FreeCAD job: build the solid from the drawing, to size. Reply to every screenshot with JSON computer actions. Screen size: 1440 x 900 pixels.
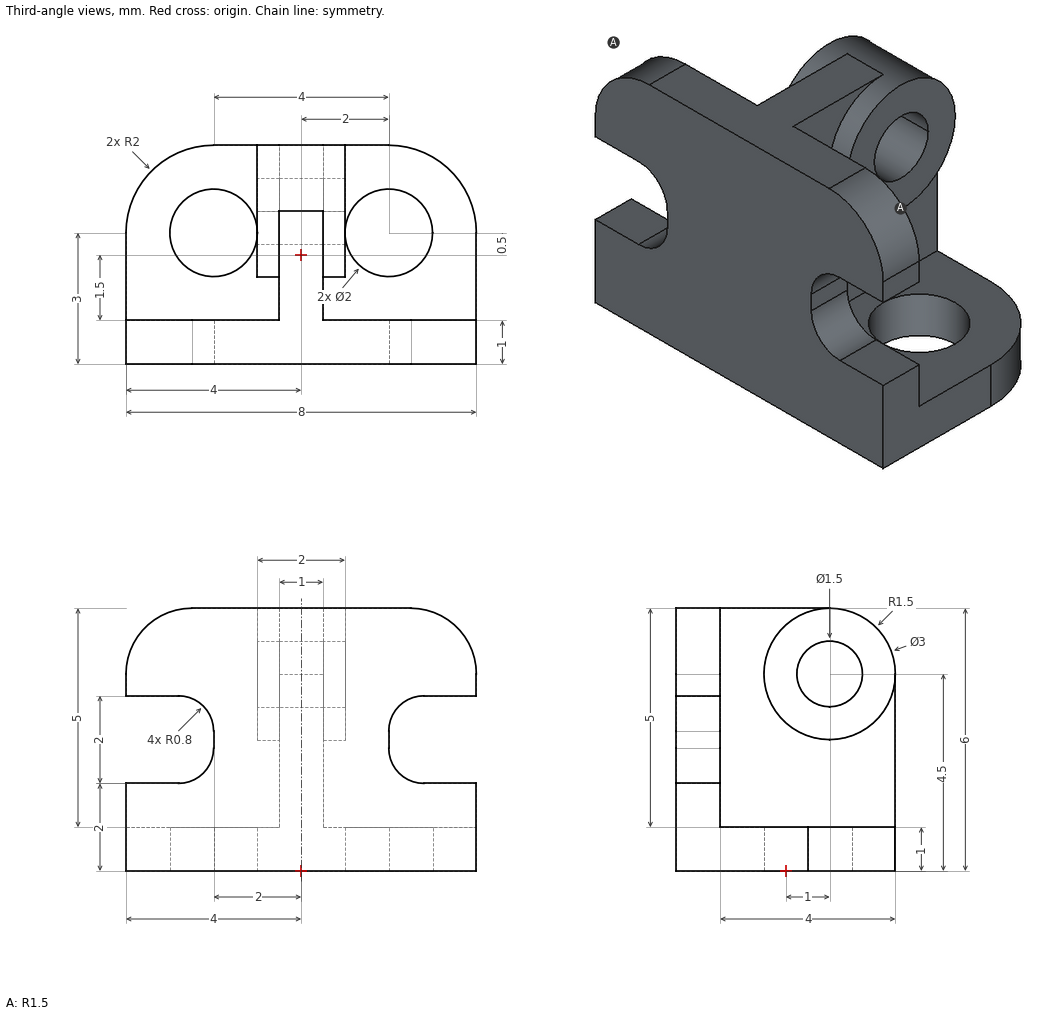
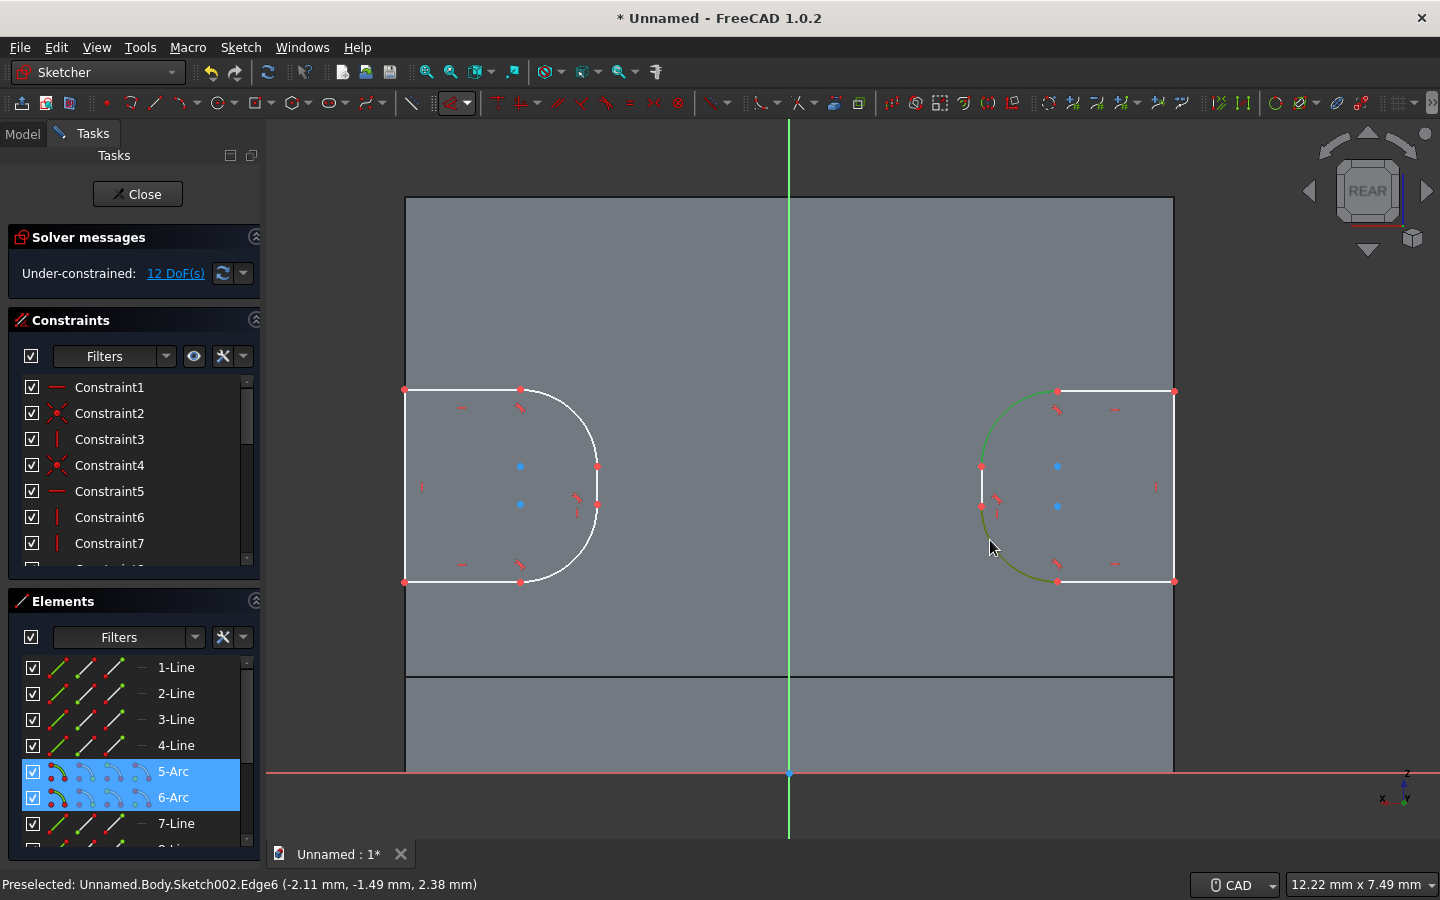
{"action": "left_click", "coordinate": [589, 432]}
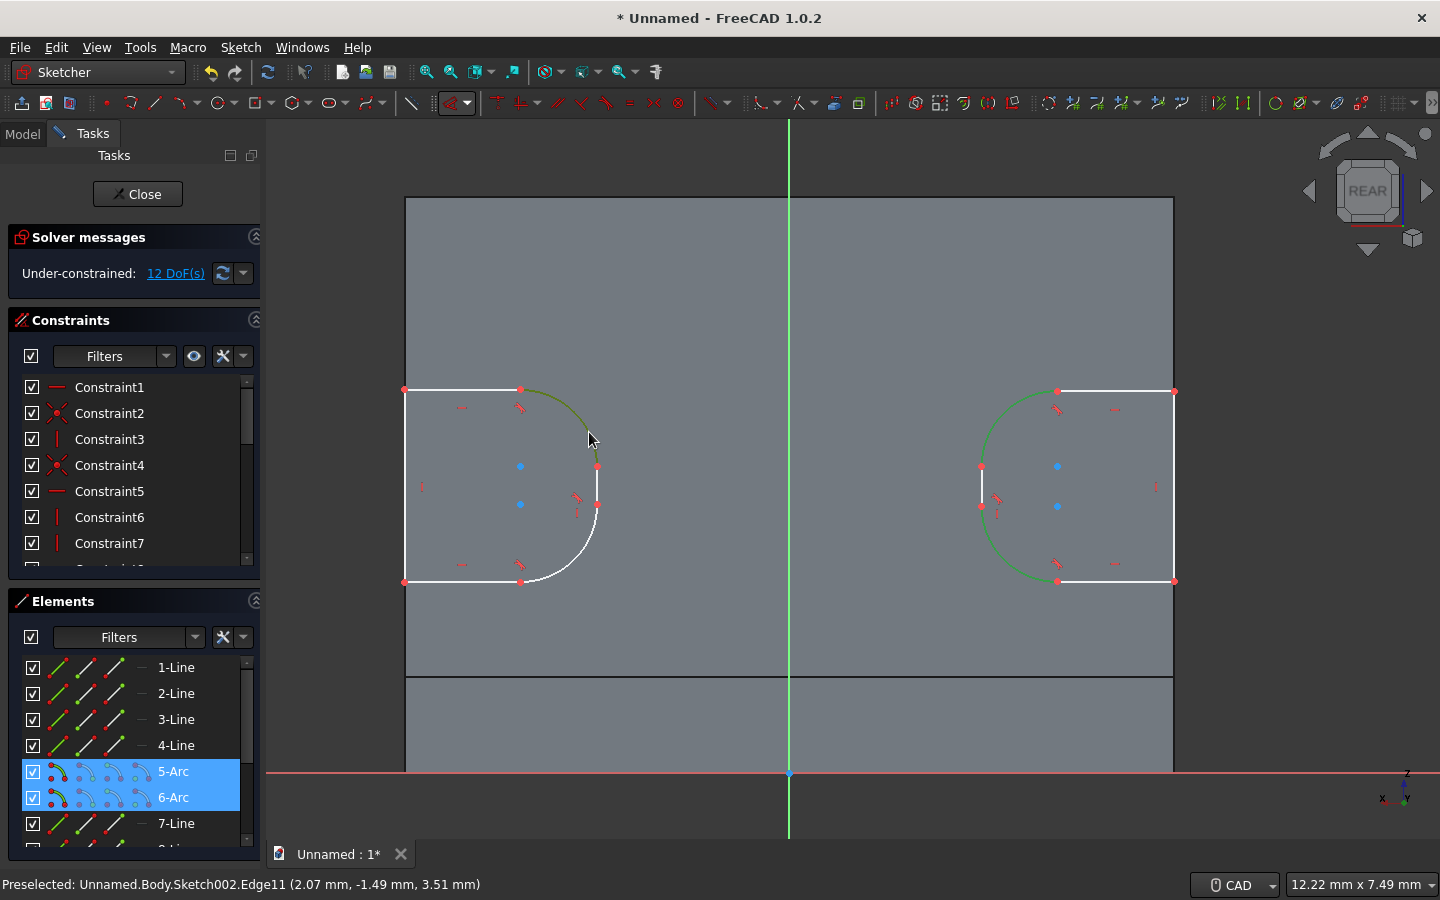
{"action": "left_click", "coordinate": [555, 574]}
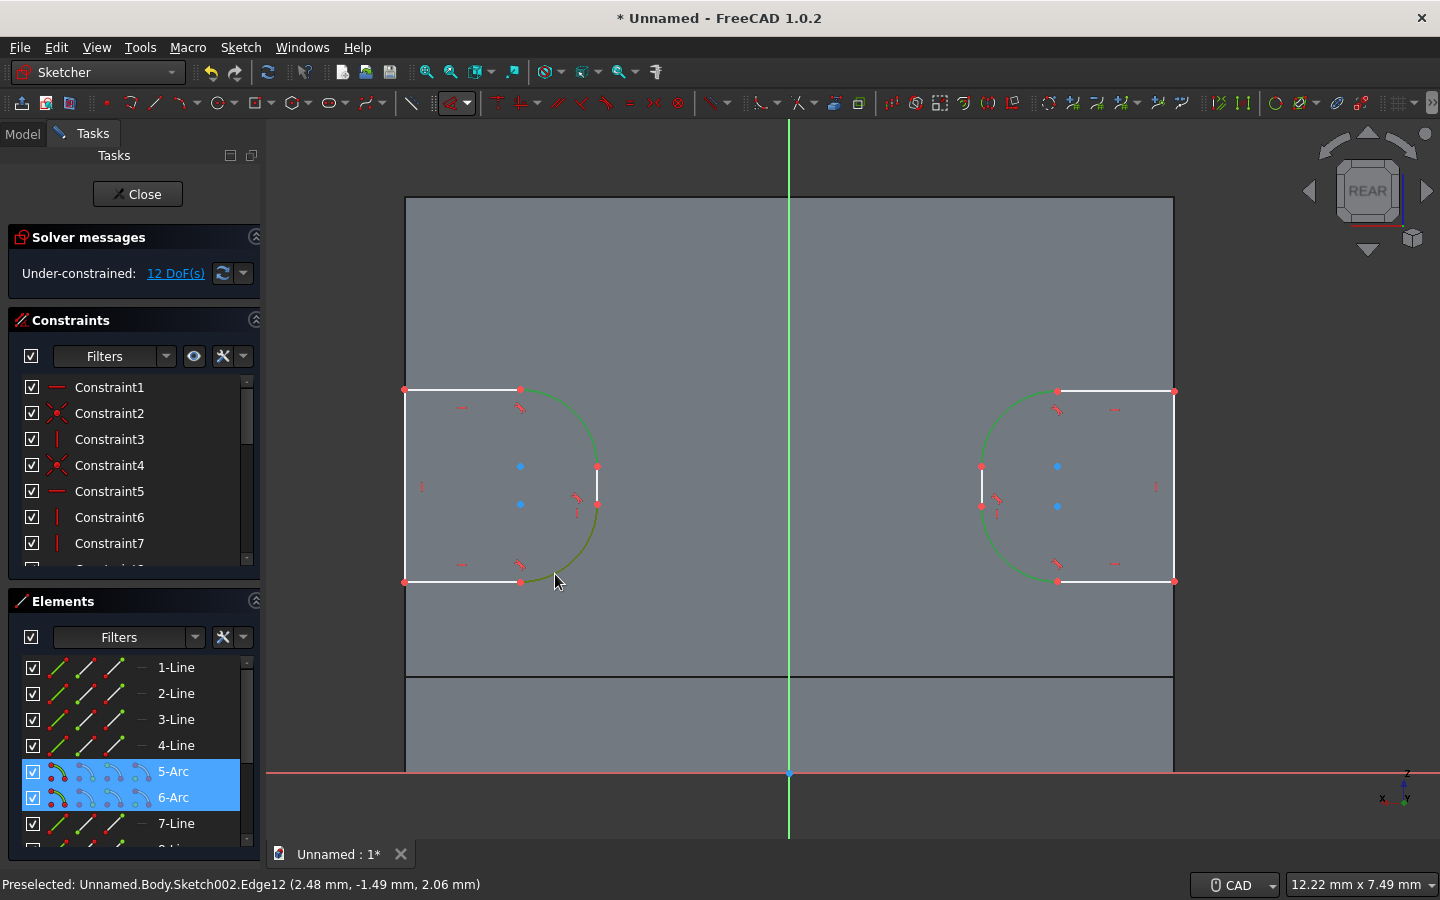
{"action": "left_click", "coordinate": [630, 104]}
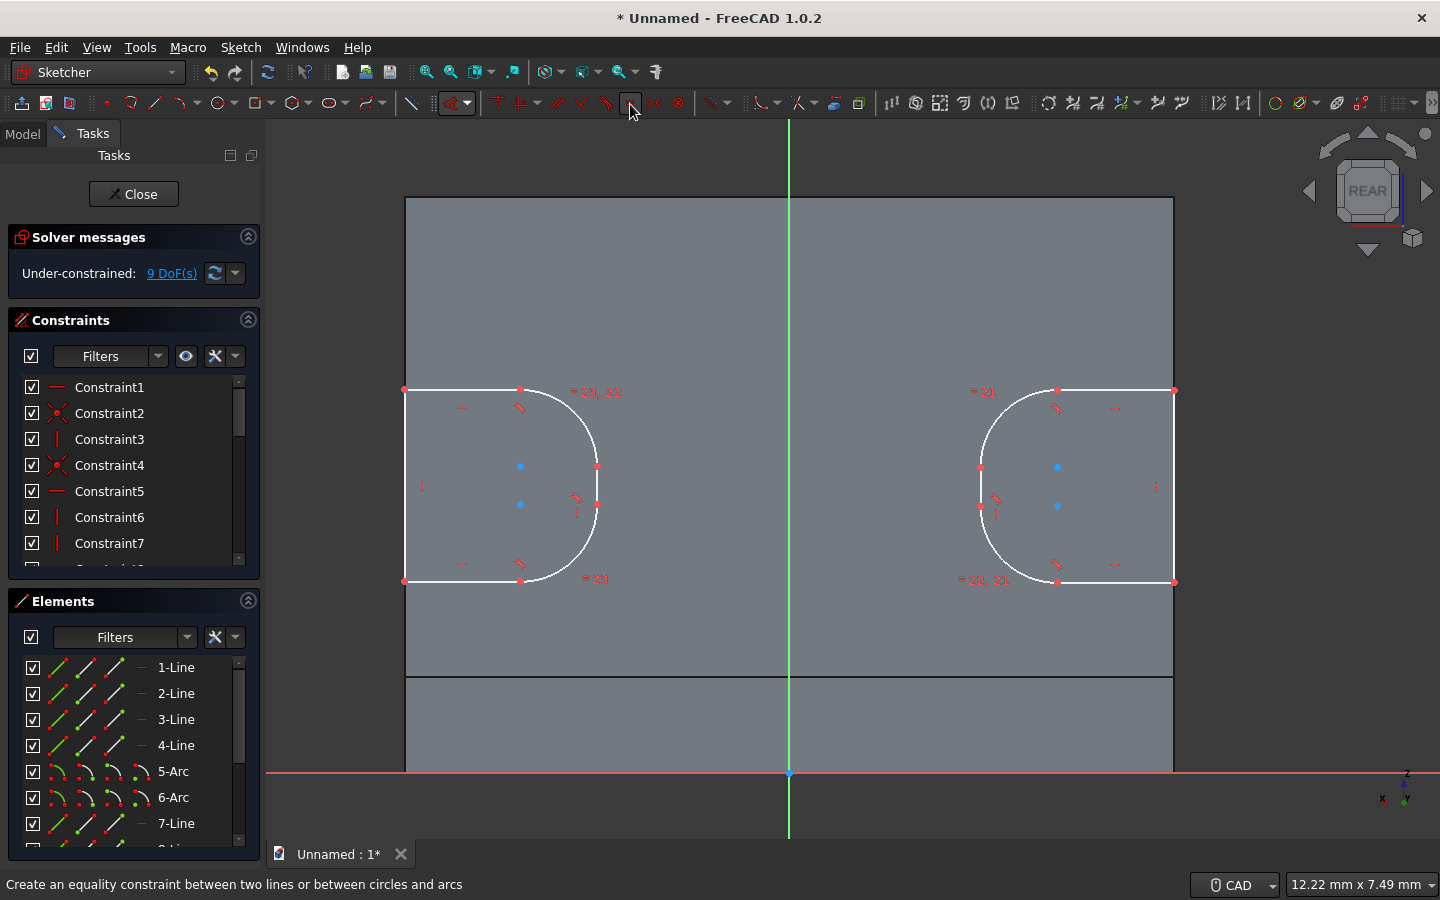
{"action": "left_click", "coordinate": [1058, 467]}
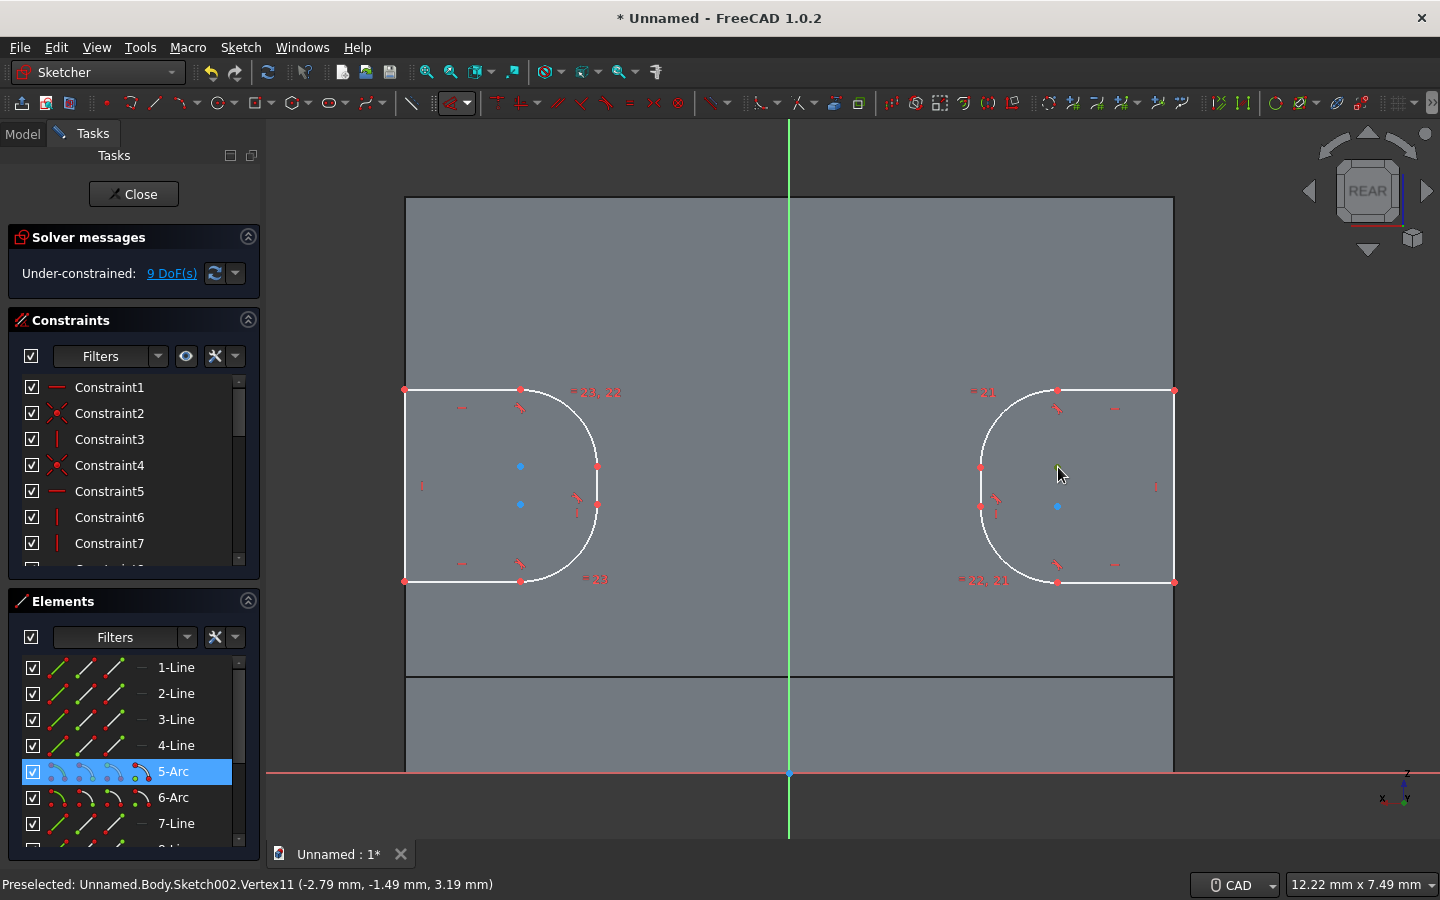
{"action": "left_click", "coordinate": [520, 467]}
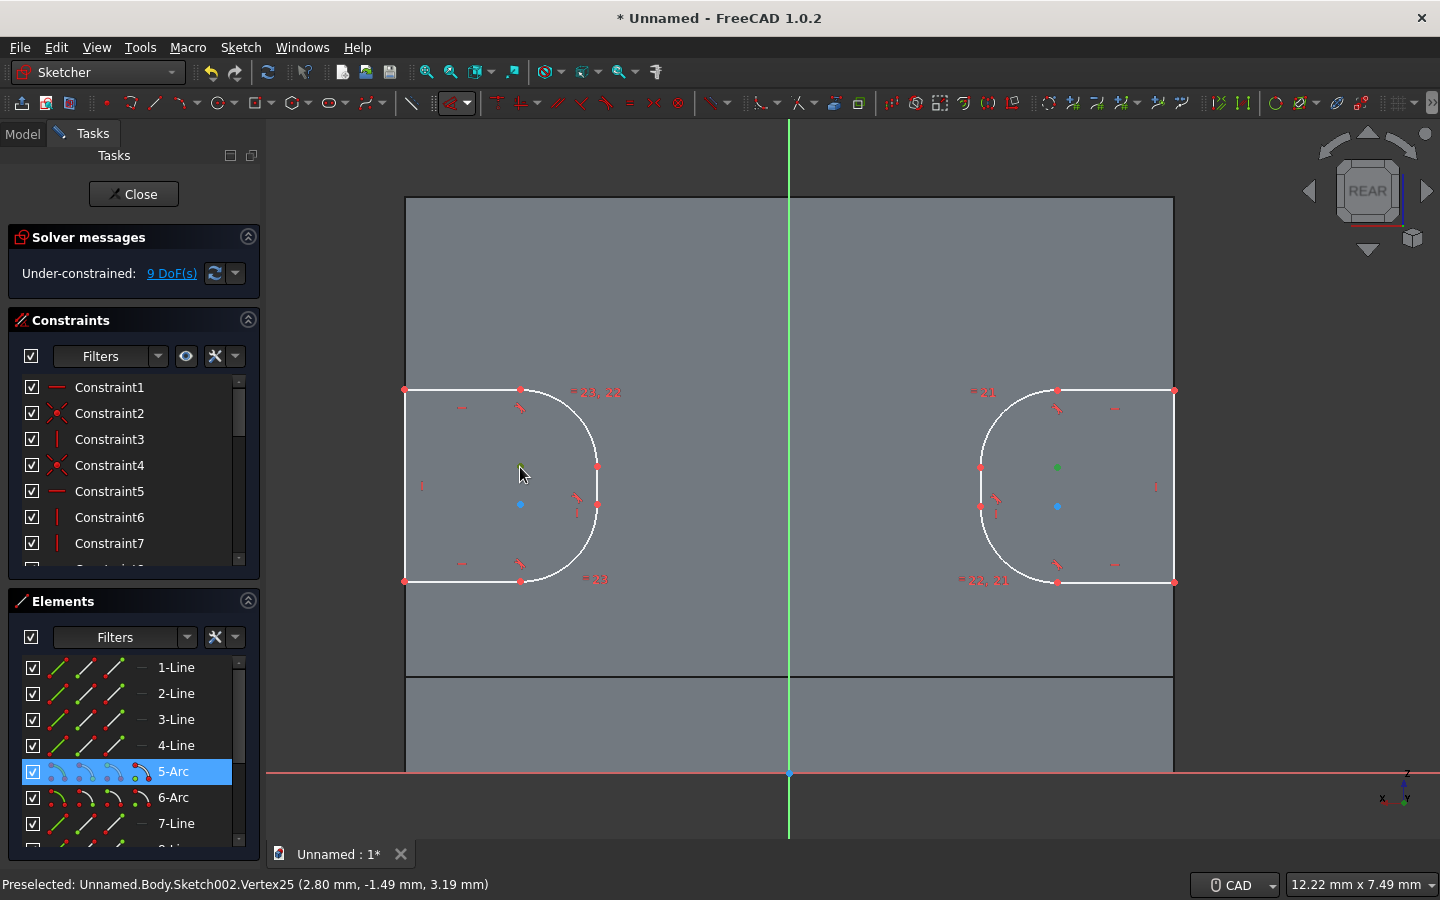
{"action": "left_click", "coordinate": [789, 716]}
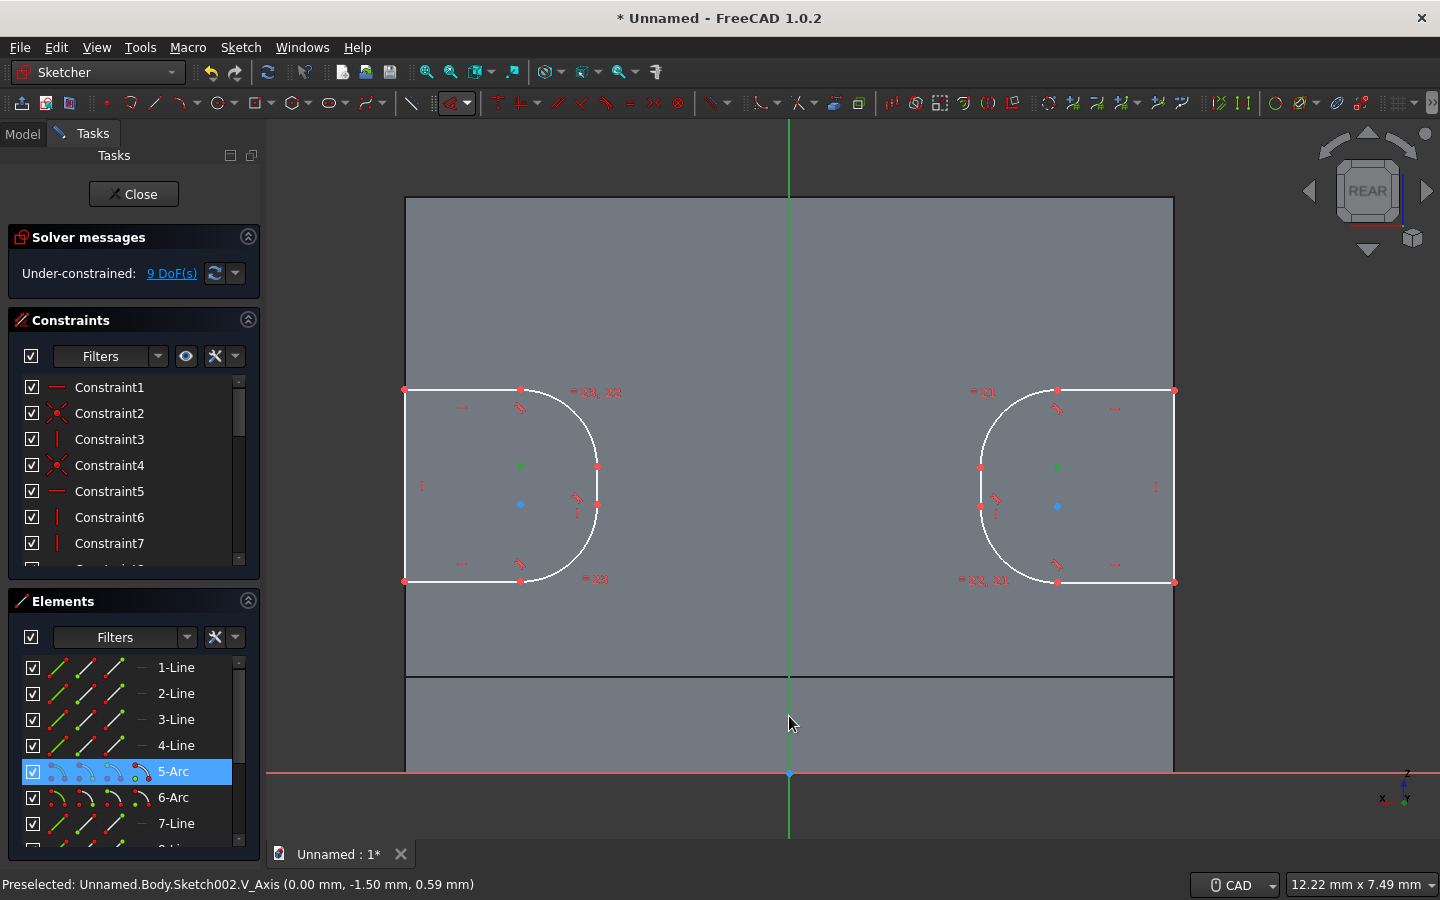
{"action": "left_click", "coordinate": [654, 104]}